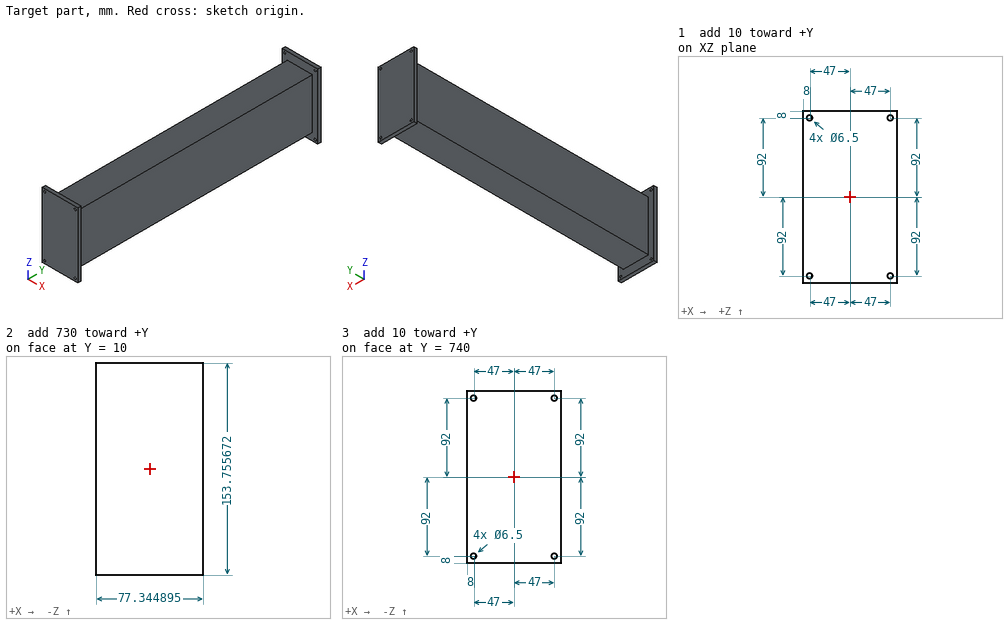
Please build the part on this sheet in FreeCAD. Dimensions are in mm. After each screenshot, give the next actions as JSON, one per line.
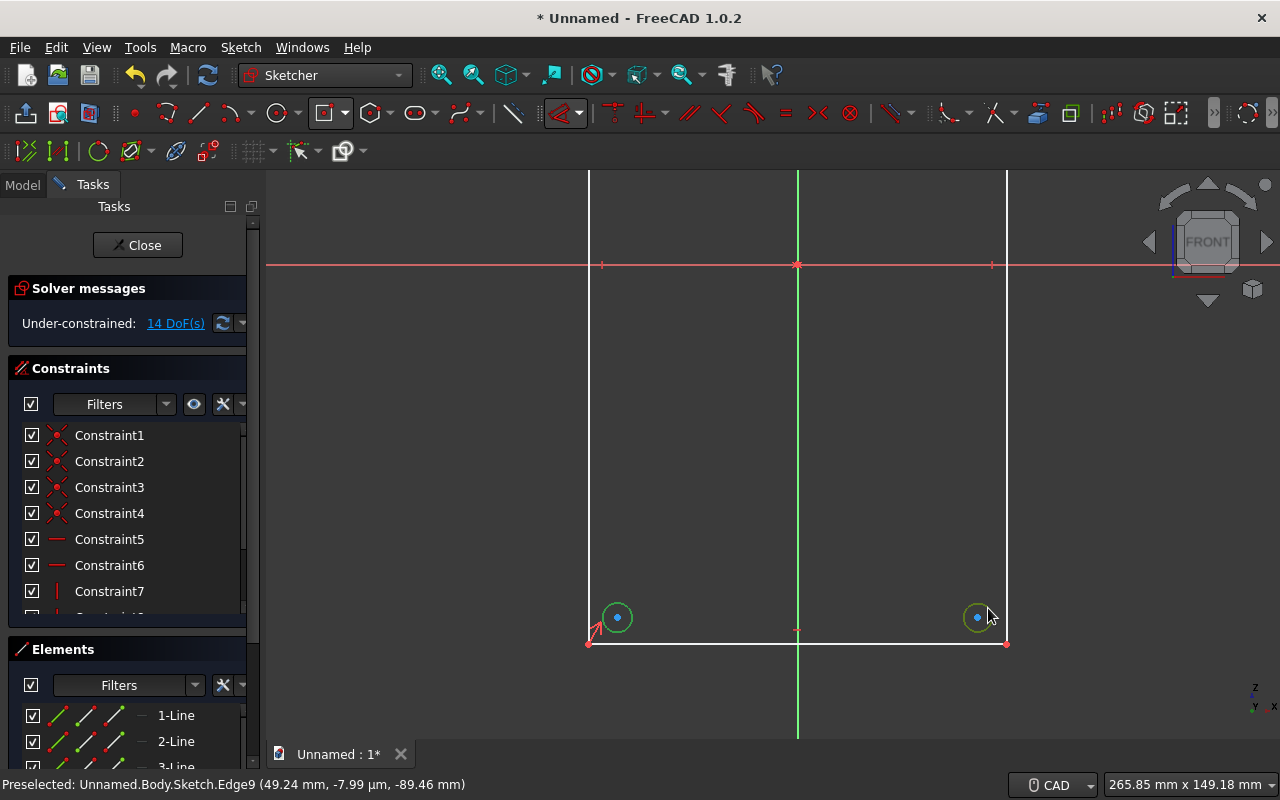
{"action": "left_click", "coordinate": [786, 114]}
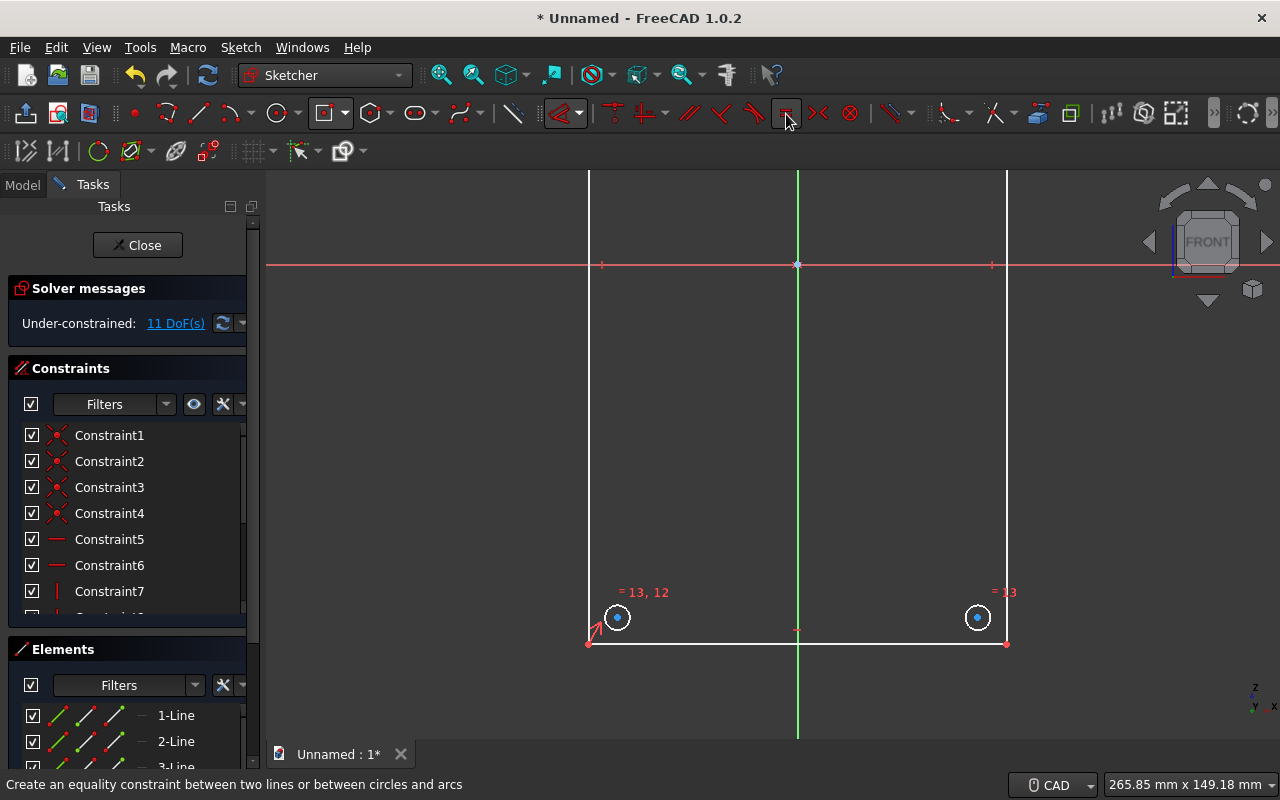
{"action": "left_click", "coordinate": [560, 114]}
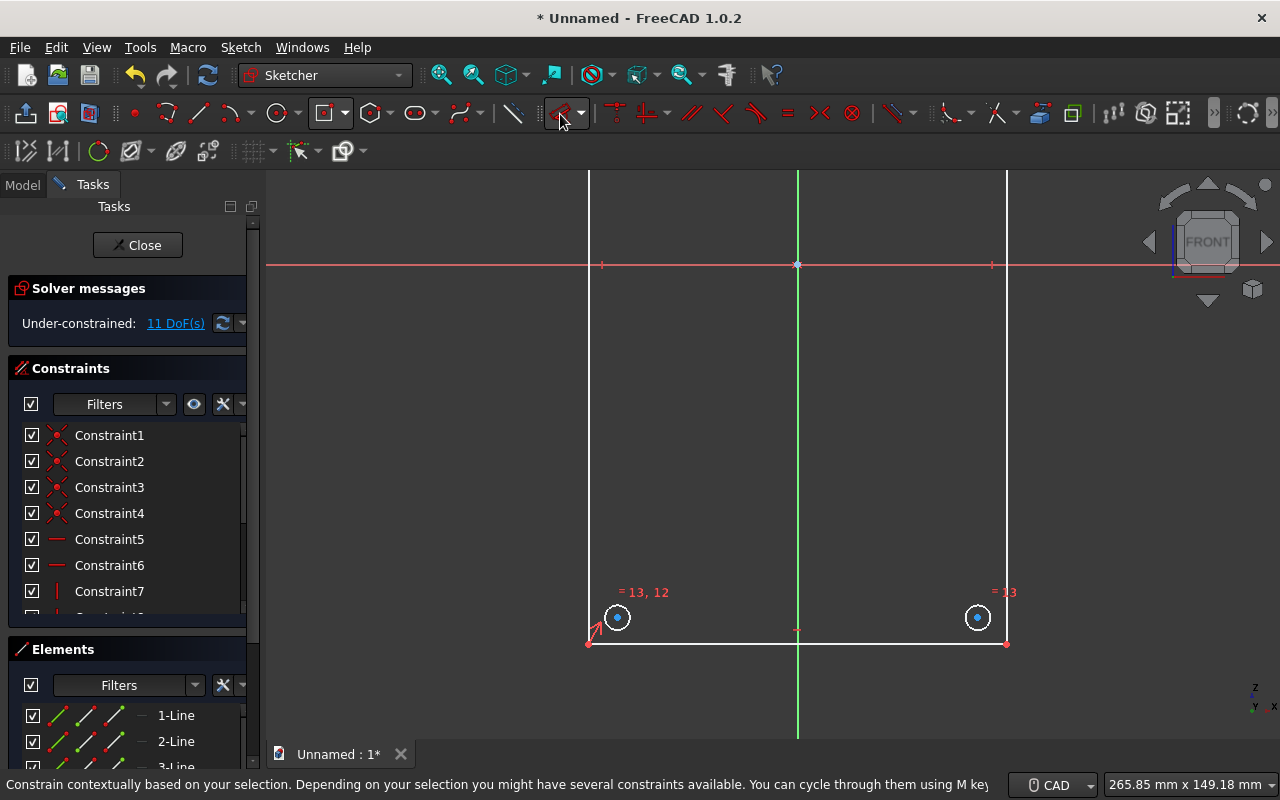
{"action": "scroll", "coordinate": [628, 609], "scroll_direction": "down", "scroll_amount": 4}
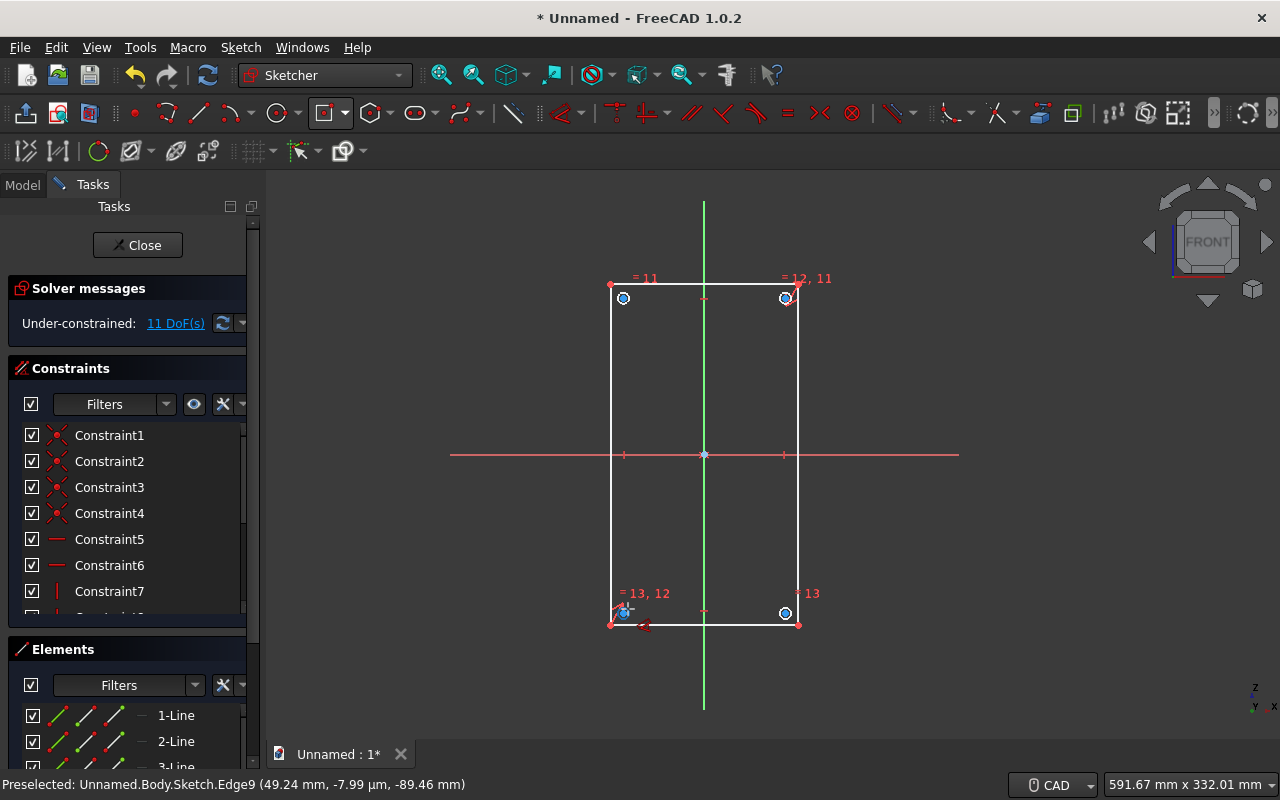
{"action": "scroll", "coordinate": [627, 294], "scroll_direction": "up", "scroll_amount": 7}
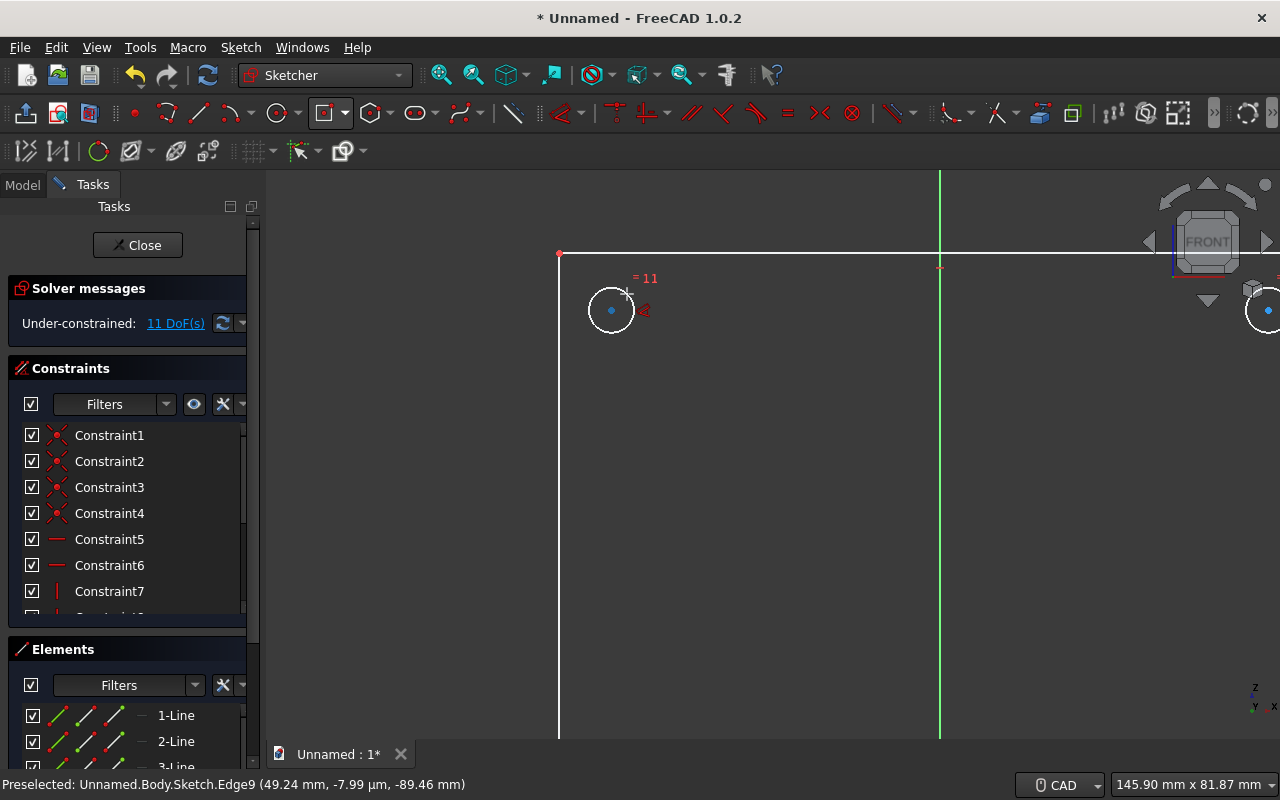
{"action": "left_click", "coordinate": [627, 294]}
{"action": "left_click", "coordinate": [649, 271]}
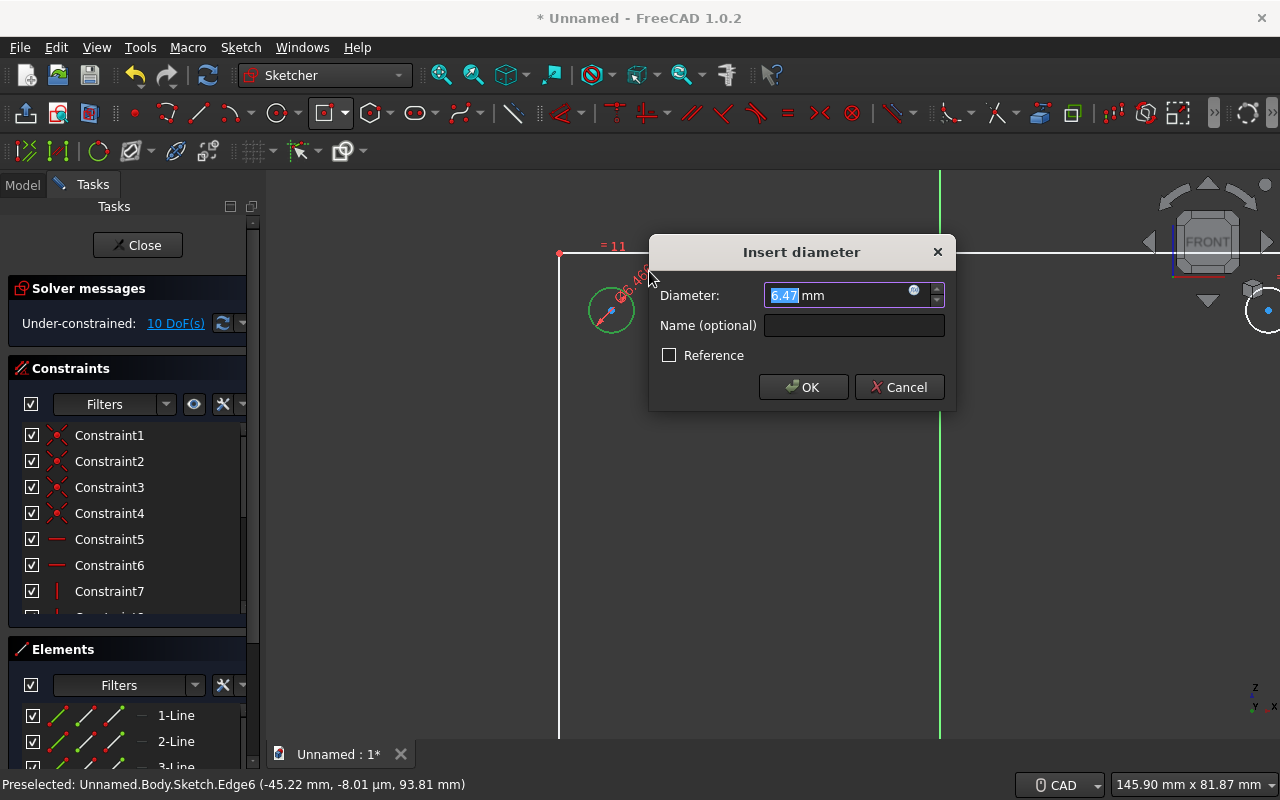
{"action": "type", "text": "6.5"}
{"action": "key", "text": "Return"}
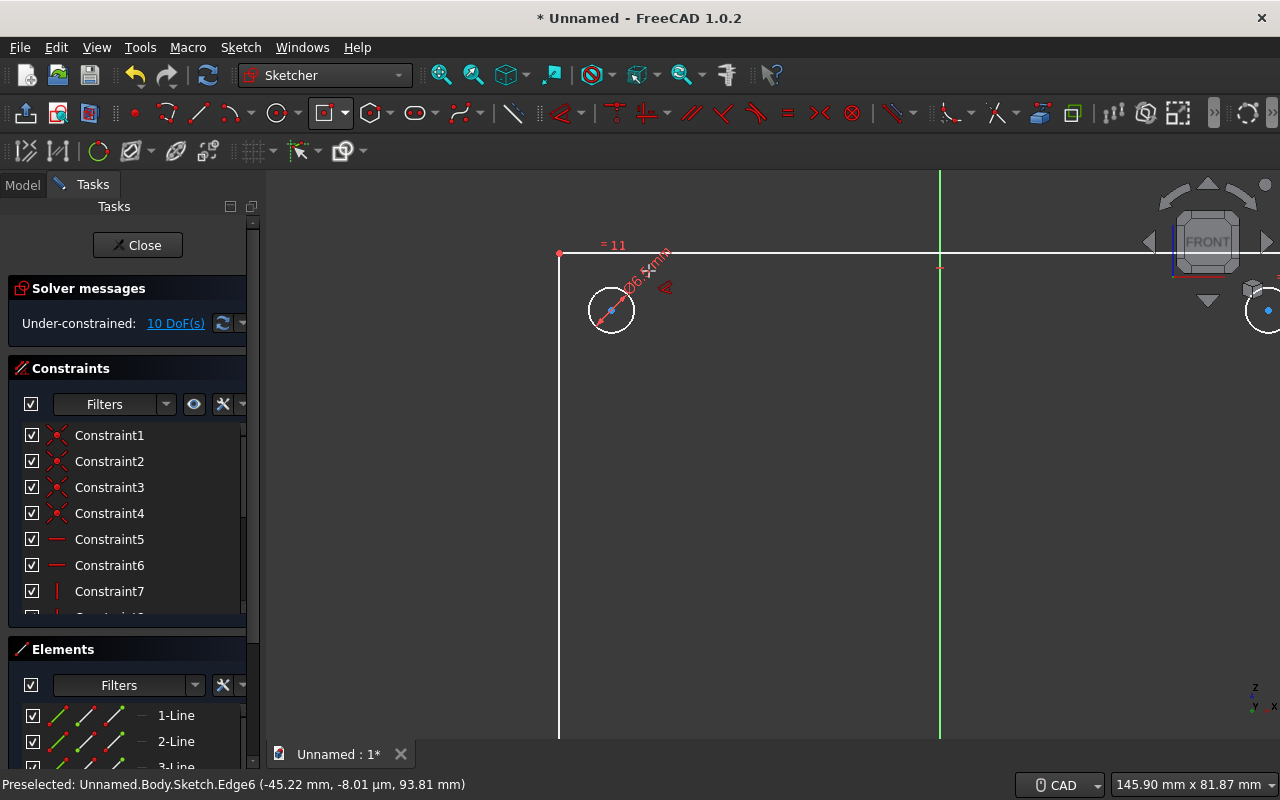
{"action": "scroll", "coordinate": [627, 294], "scroll_direction": "down", "scroll_amount": 7}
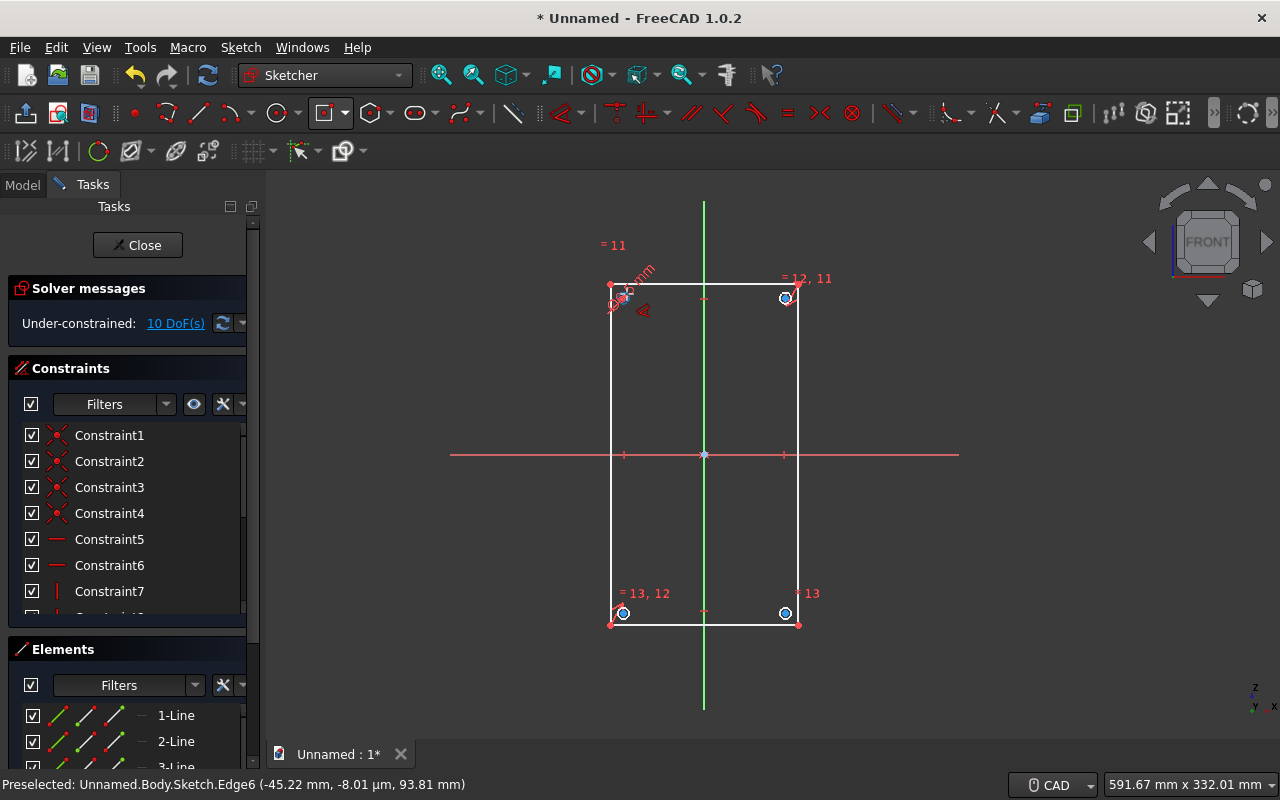
{"action": "left_click", "coordinate": [623, 298]}
{"action": "left_click", "coordinate": [664, 264]}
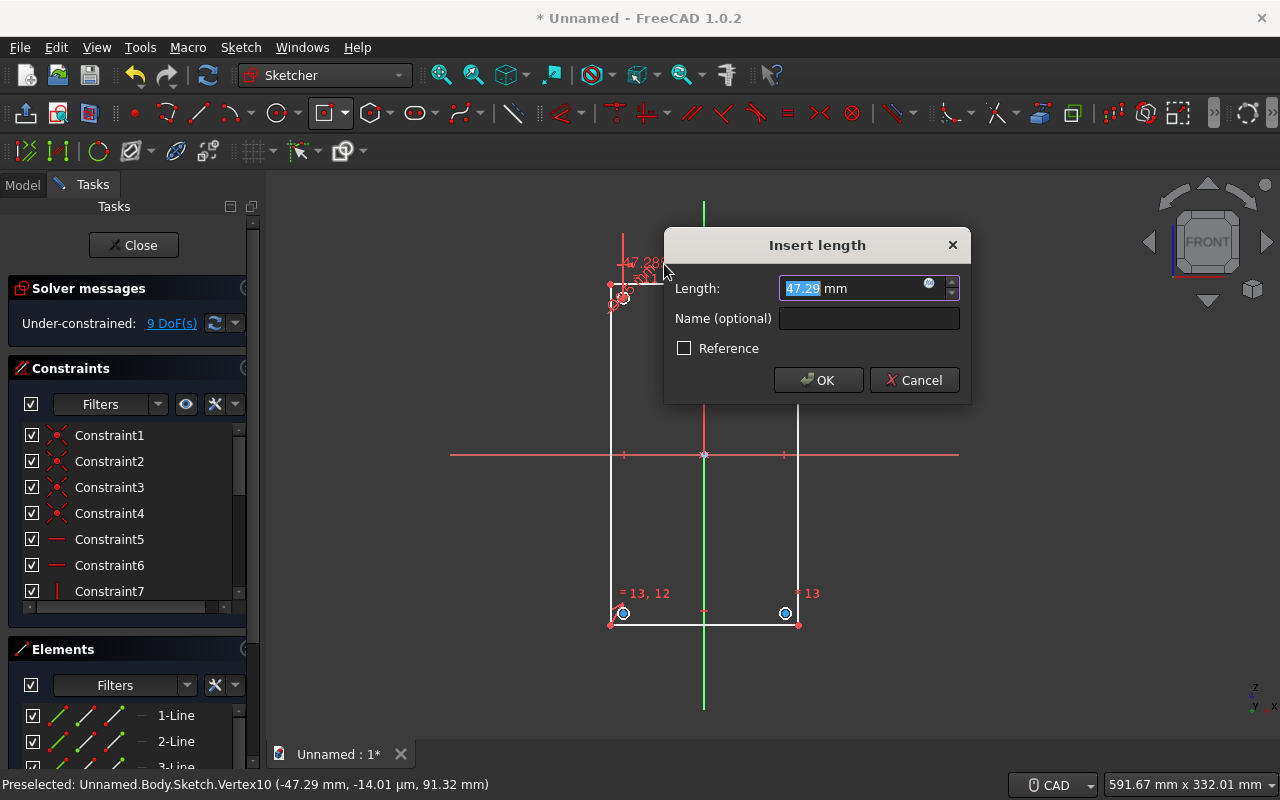
{"action": "type", "text": "47"}
{"action": "key", "text": "Return"}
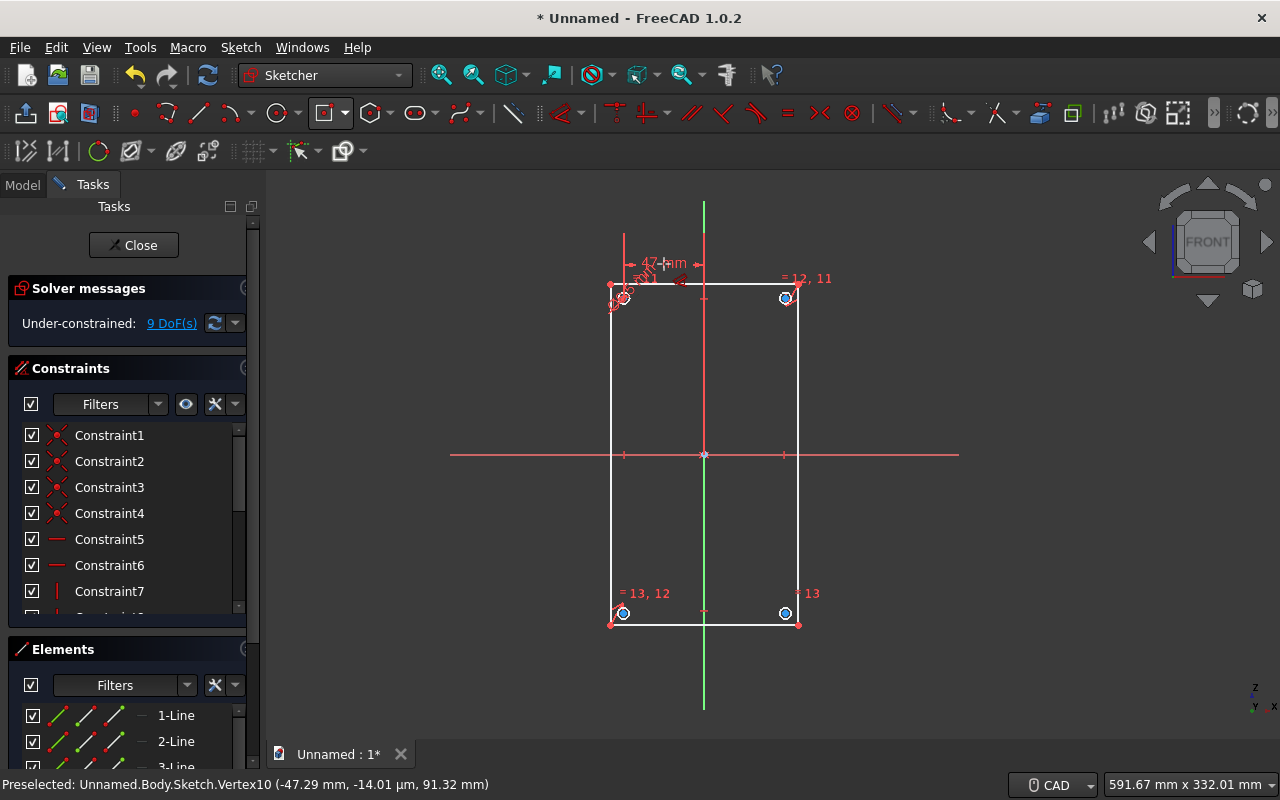
{"action": "left_click", "coordinate": [624, 298]}
{"action": "left_click", "coordinate": [590, 376]}